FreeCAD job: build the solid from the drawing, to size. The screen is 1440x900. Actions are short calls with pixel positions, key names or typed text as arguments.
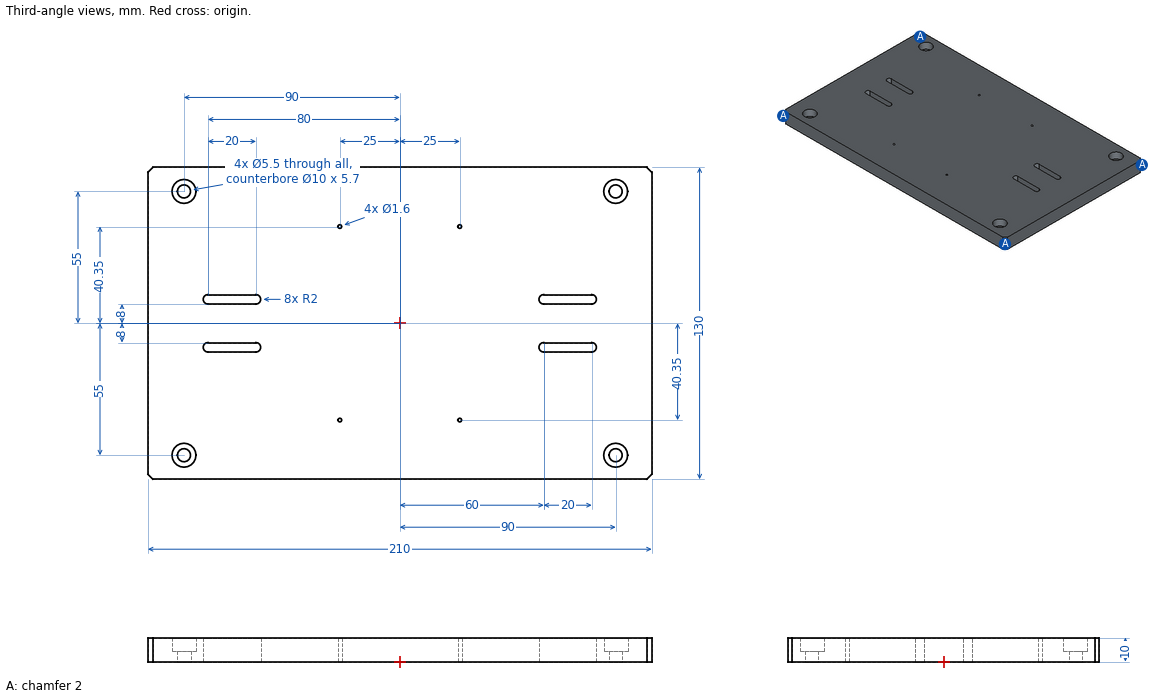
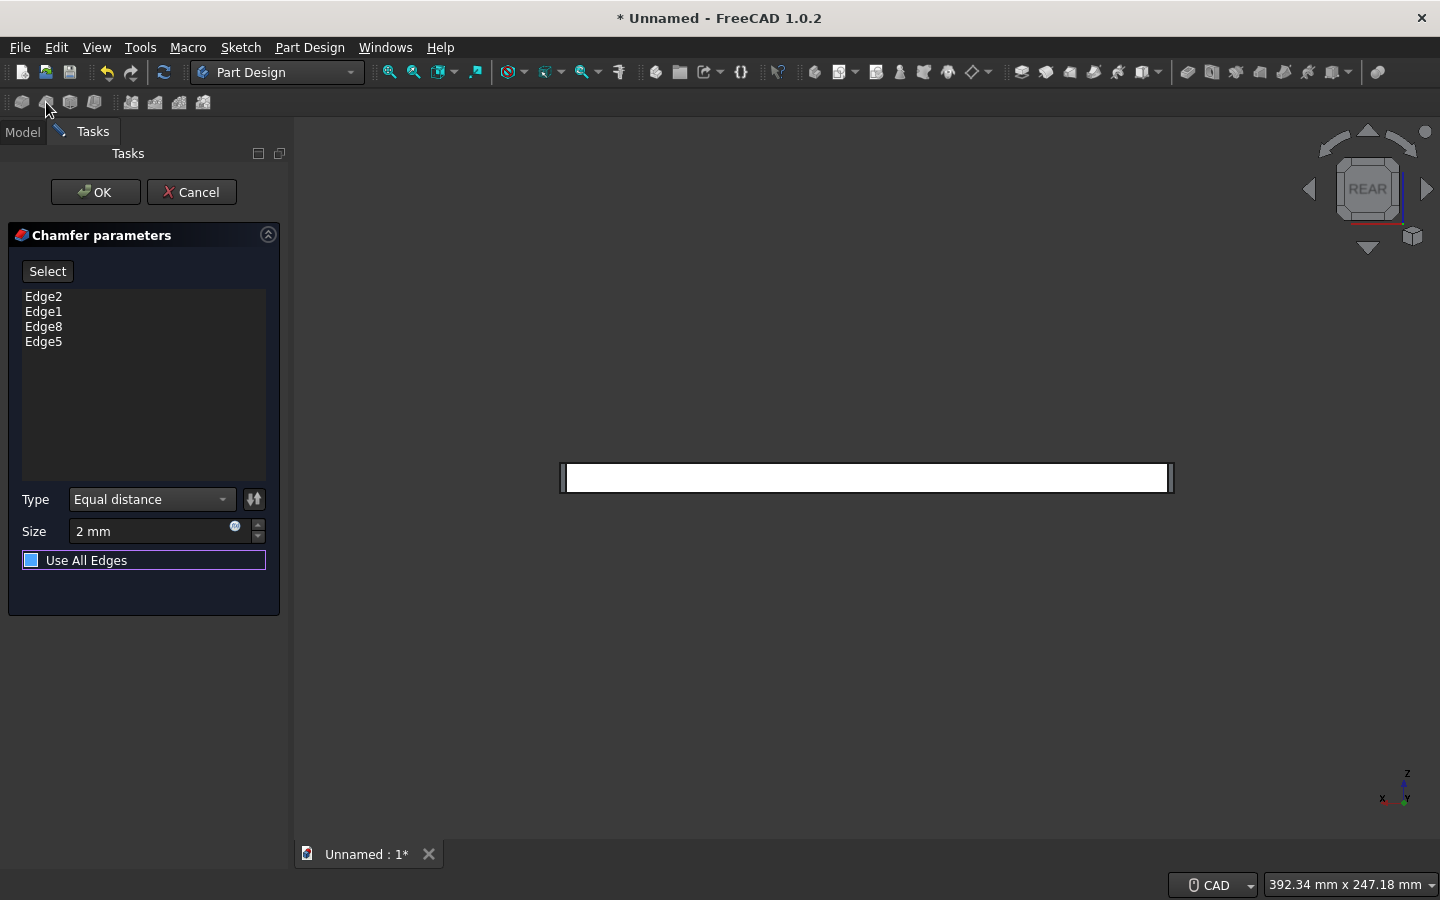
click(96, 192)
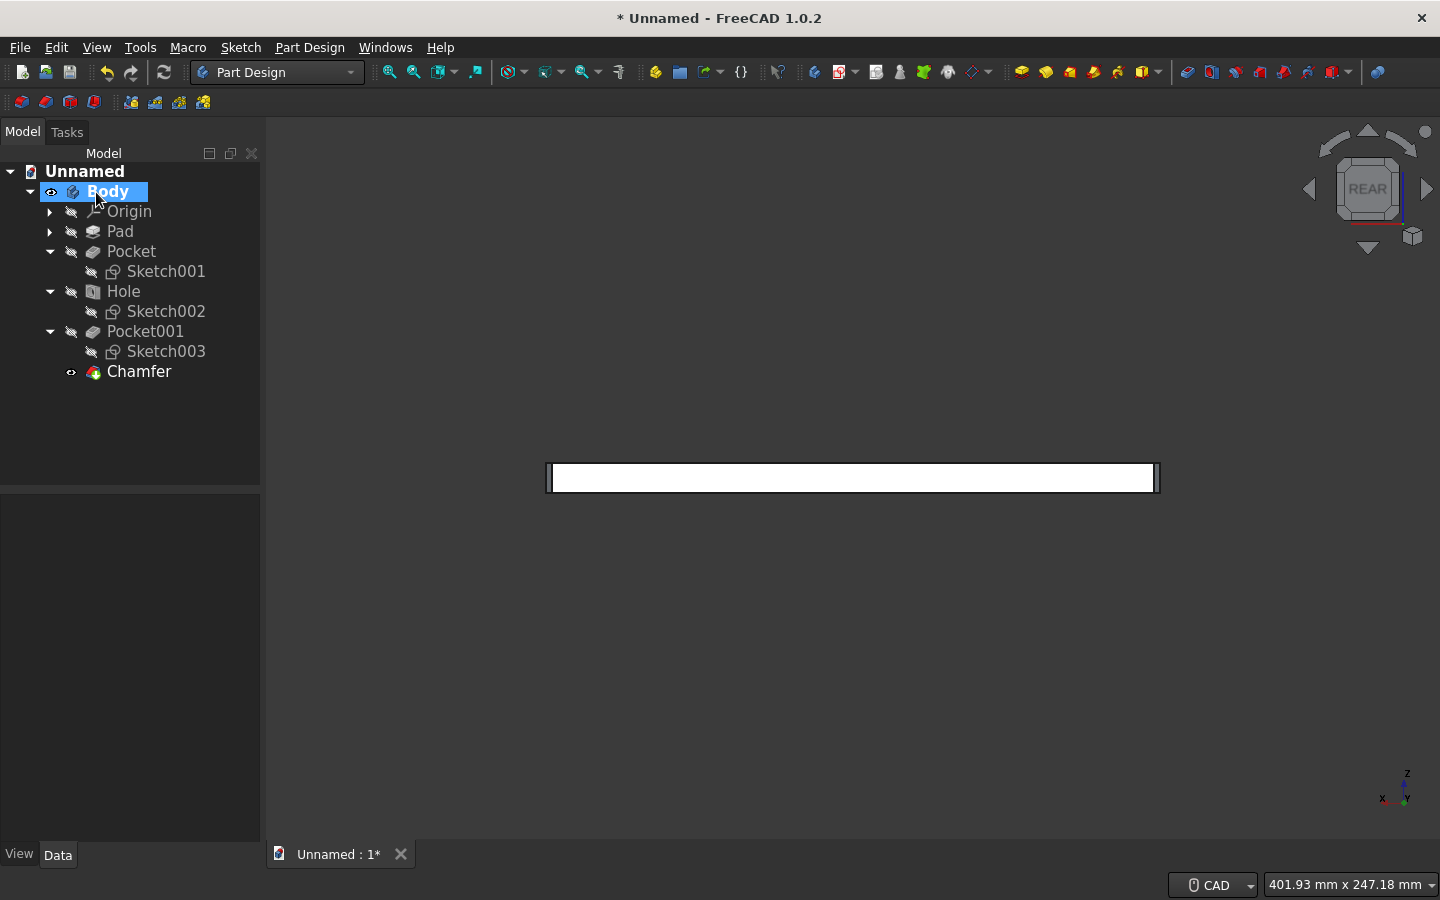
key(0)